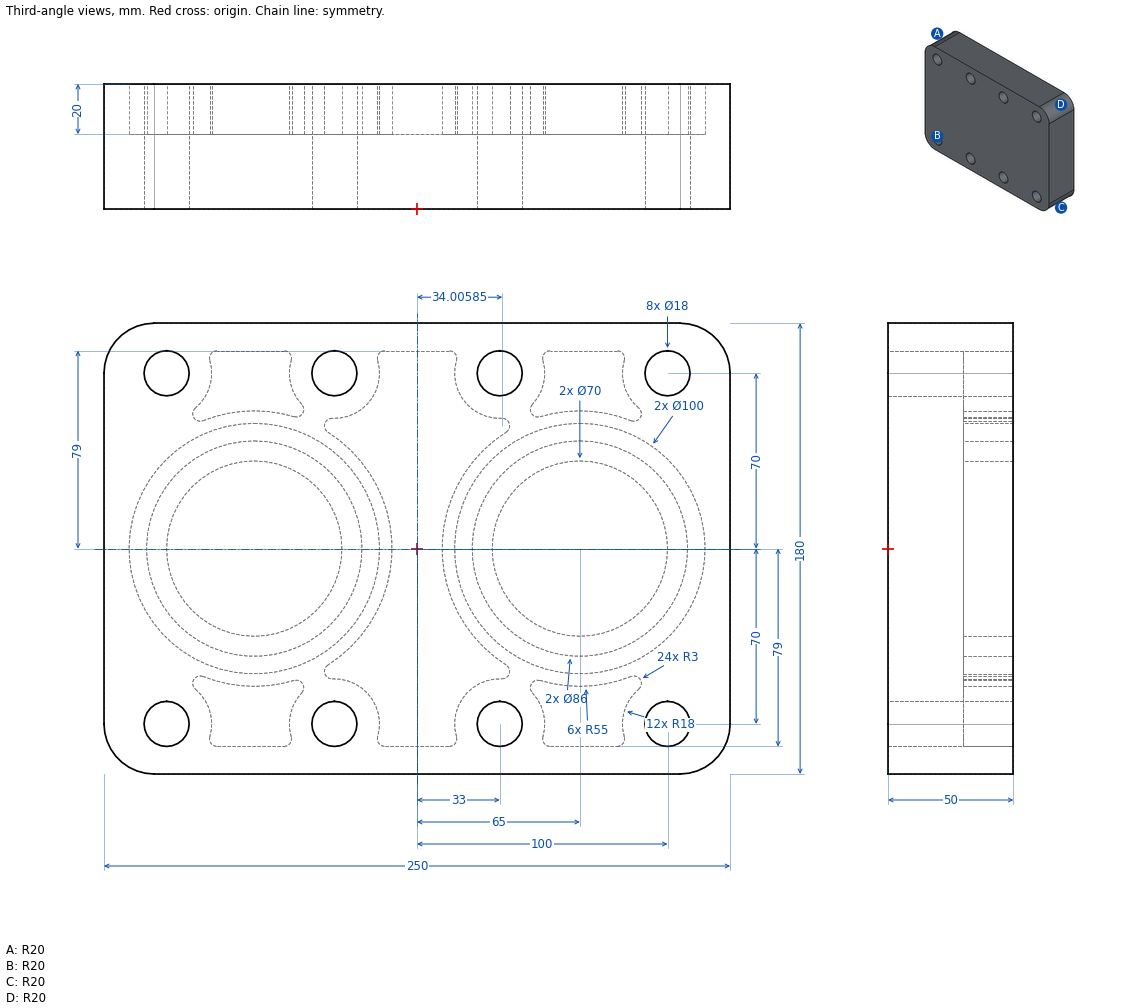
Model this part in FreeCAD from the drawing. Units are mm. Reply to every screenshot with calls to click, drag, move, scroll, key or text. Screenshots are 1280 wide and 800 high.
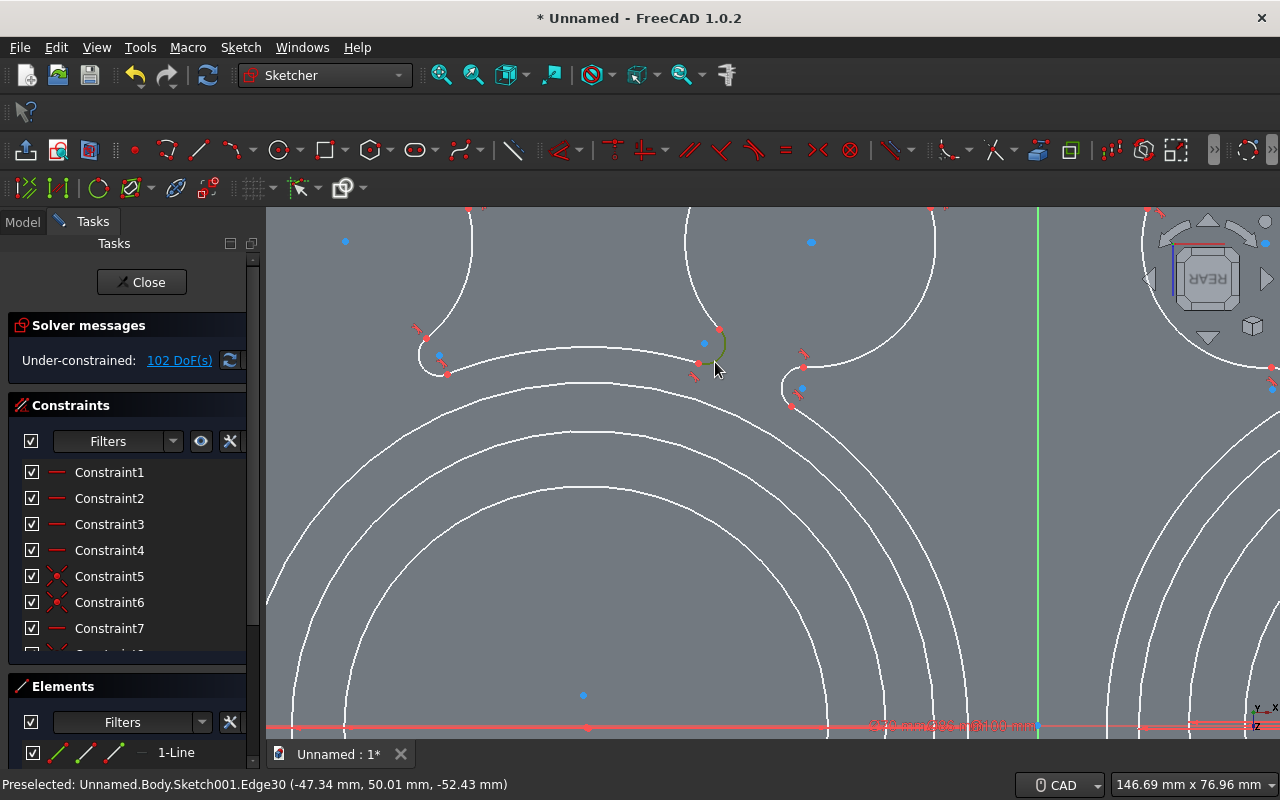
click(685, 246)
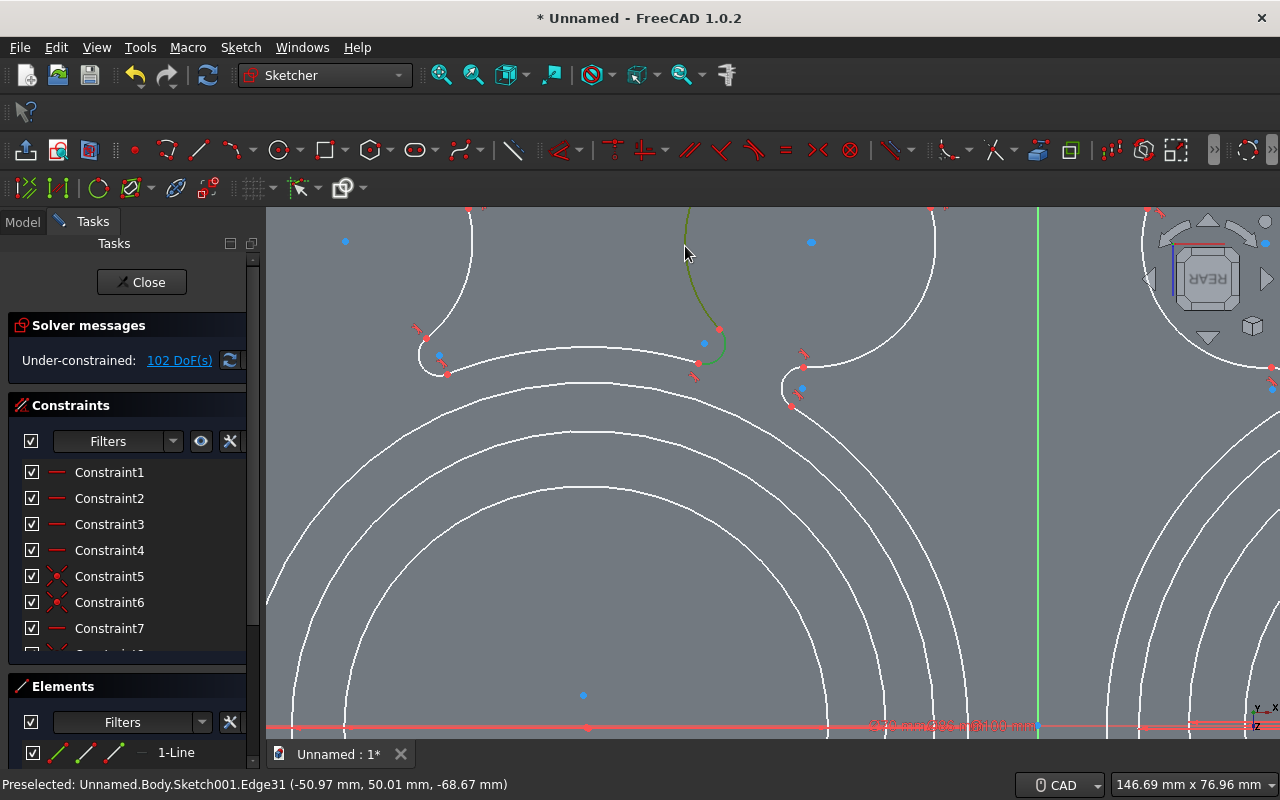
click(754, 150)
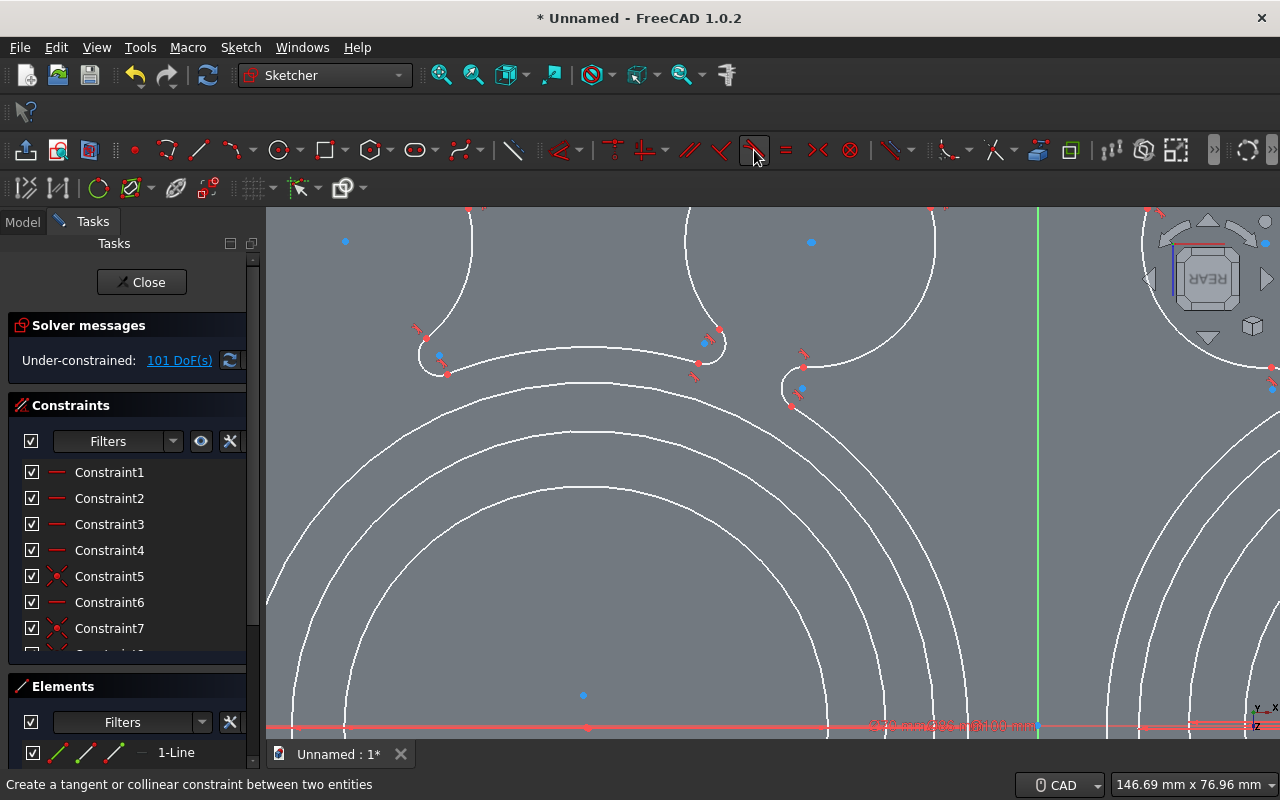
click(685, 246)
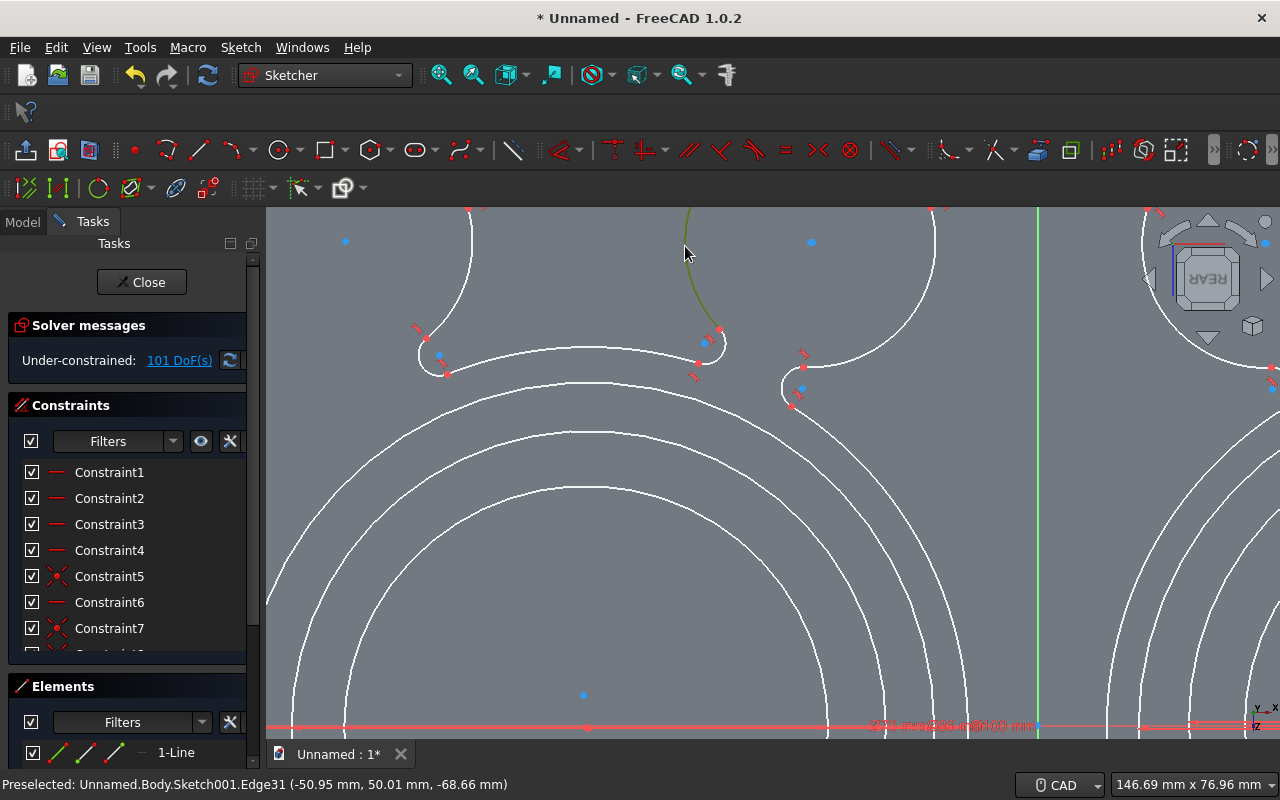
scroll(561, 364, down, 6)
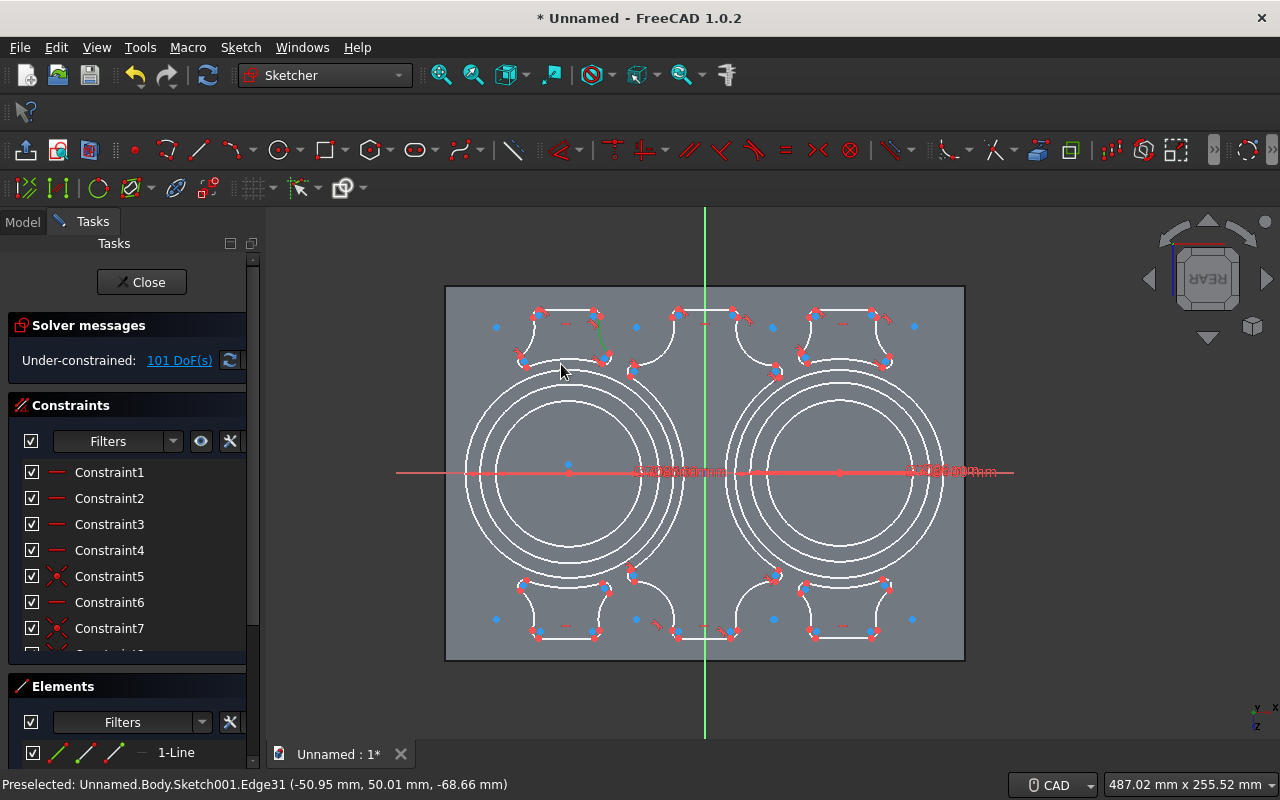
scroll(600, 314, up, 8)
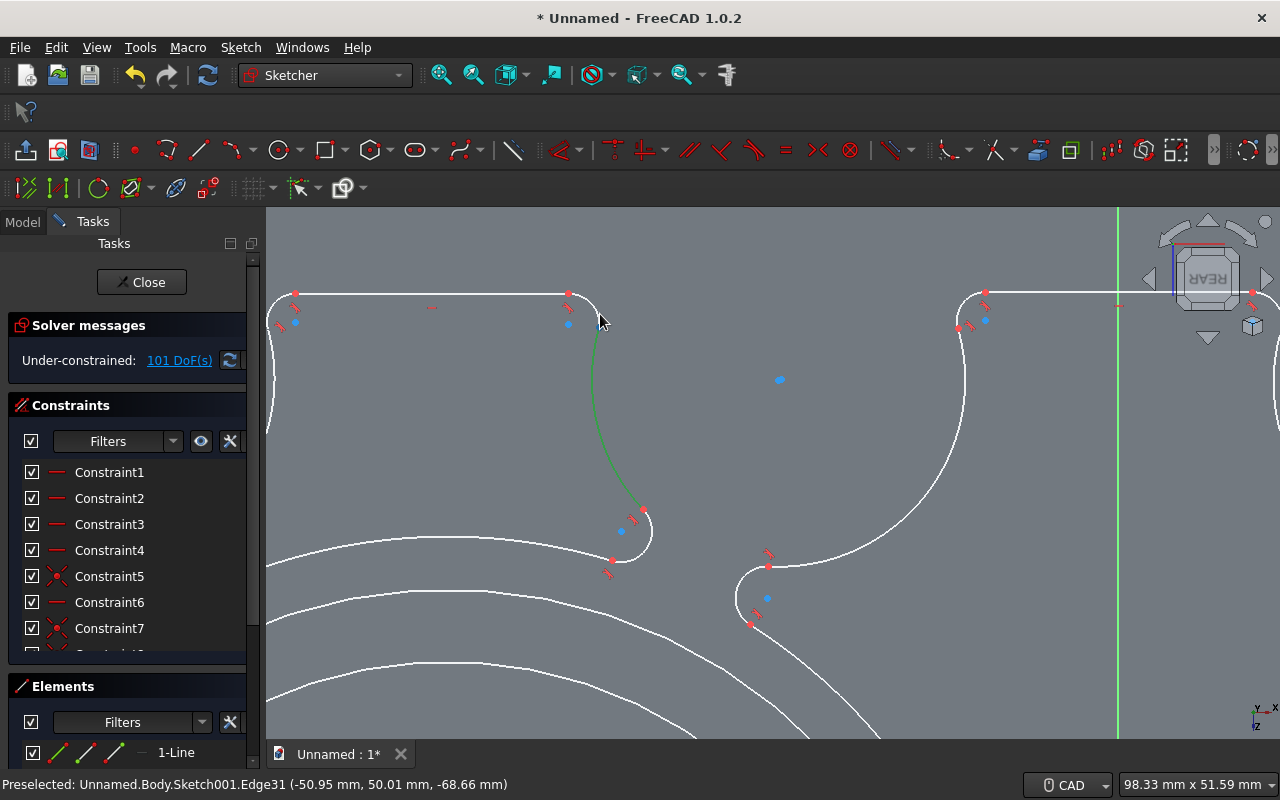
click(597, 312)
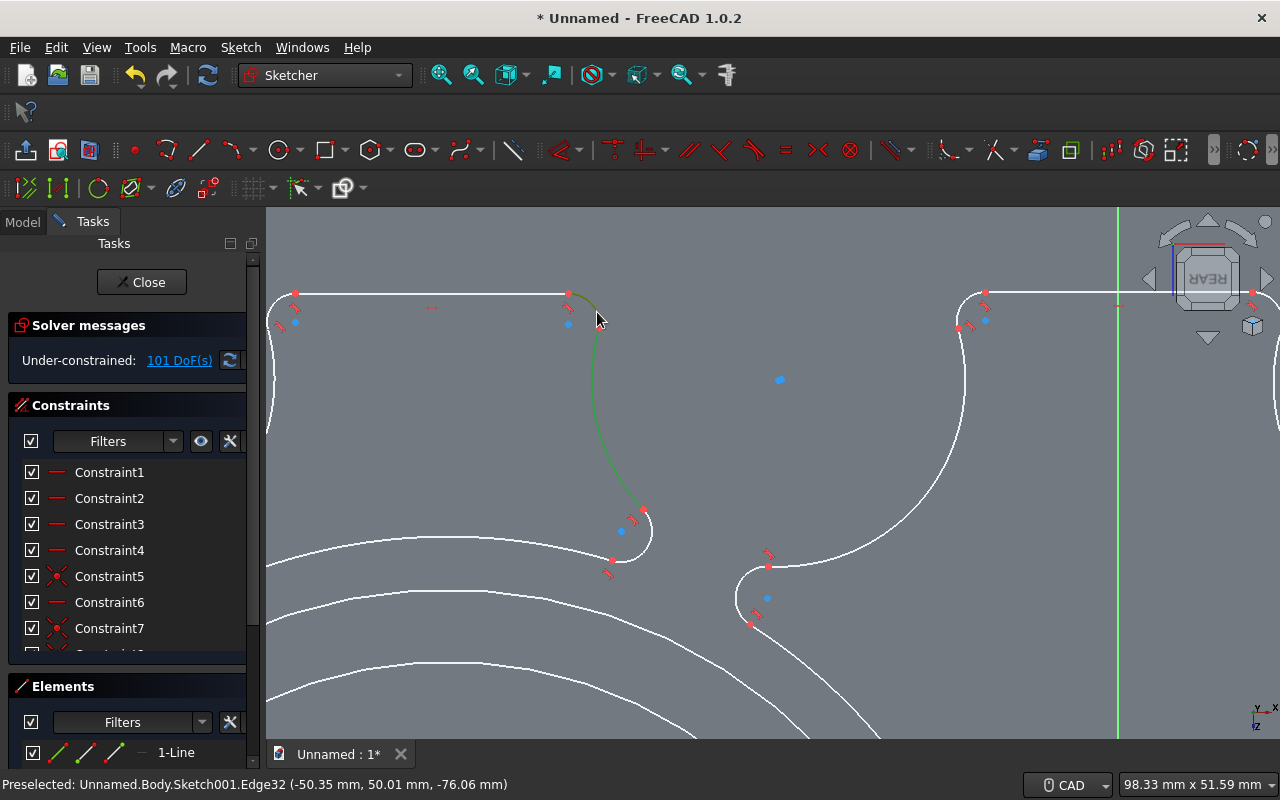
click(754, 150)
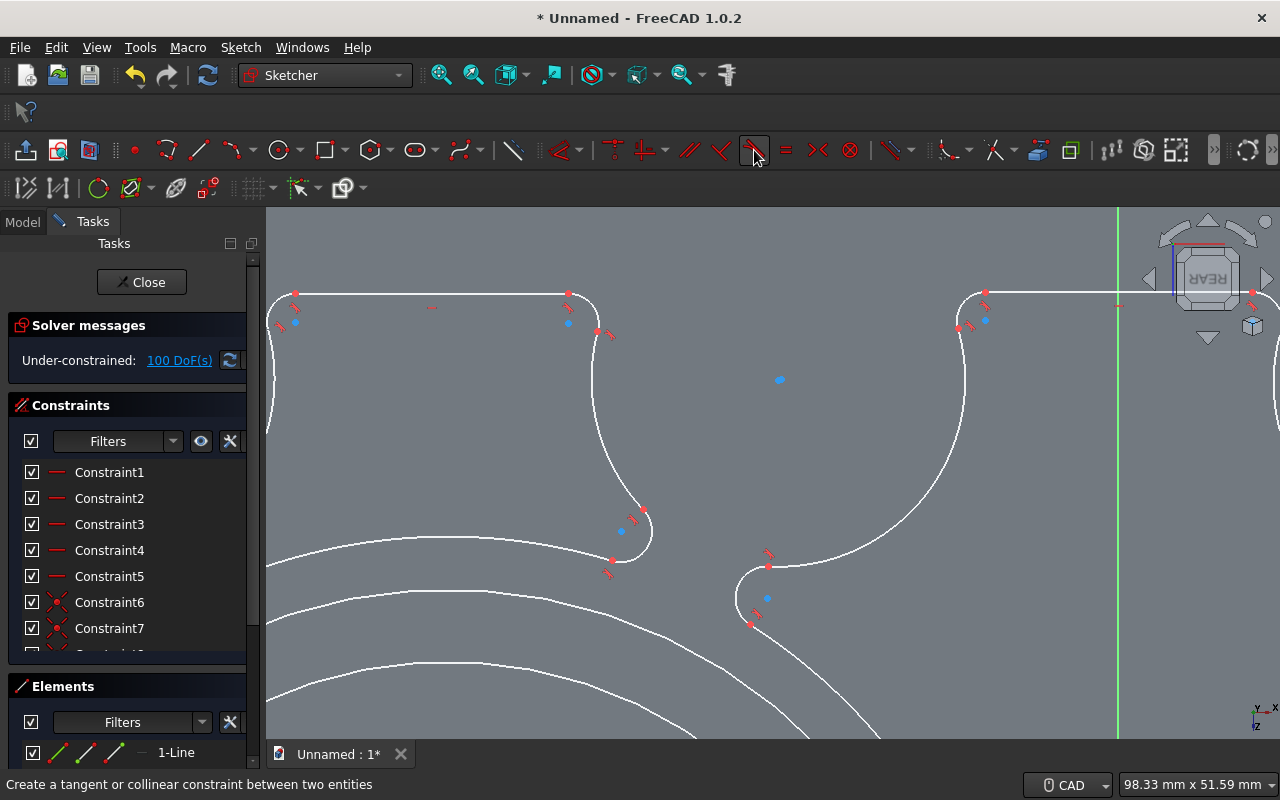
scroll(600, 314, down, 8)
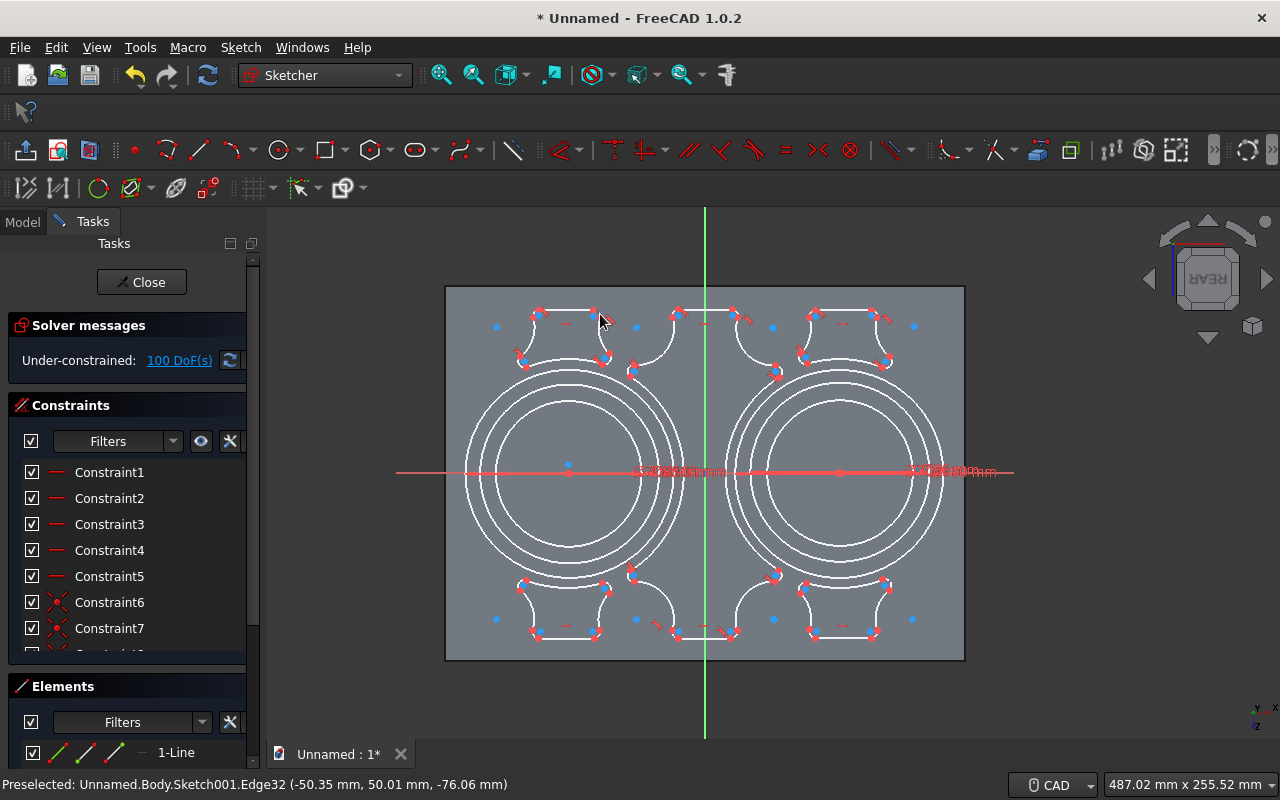
click(555, 639)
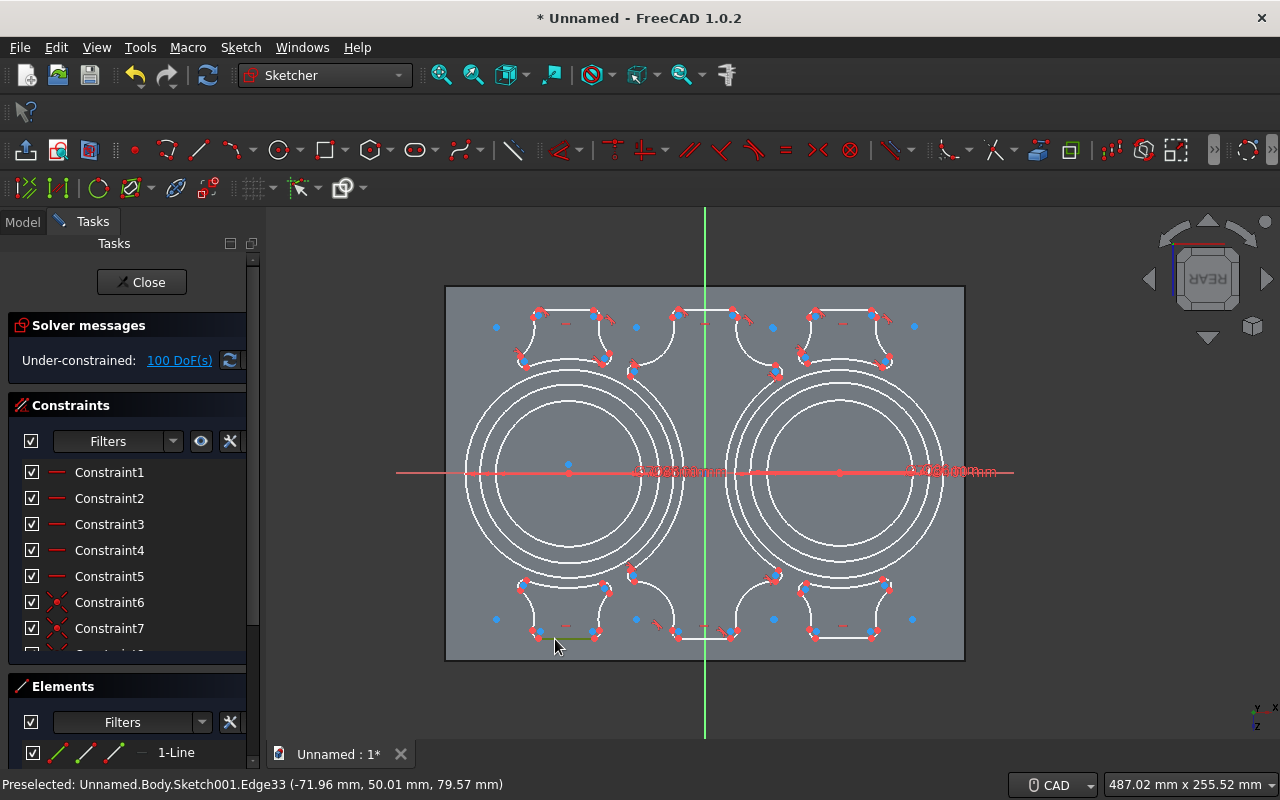
scroll(599, 636, up, 5)